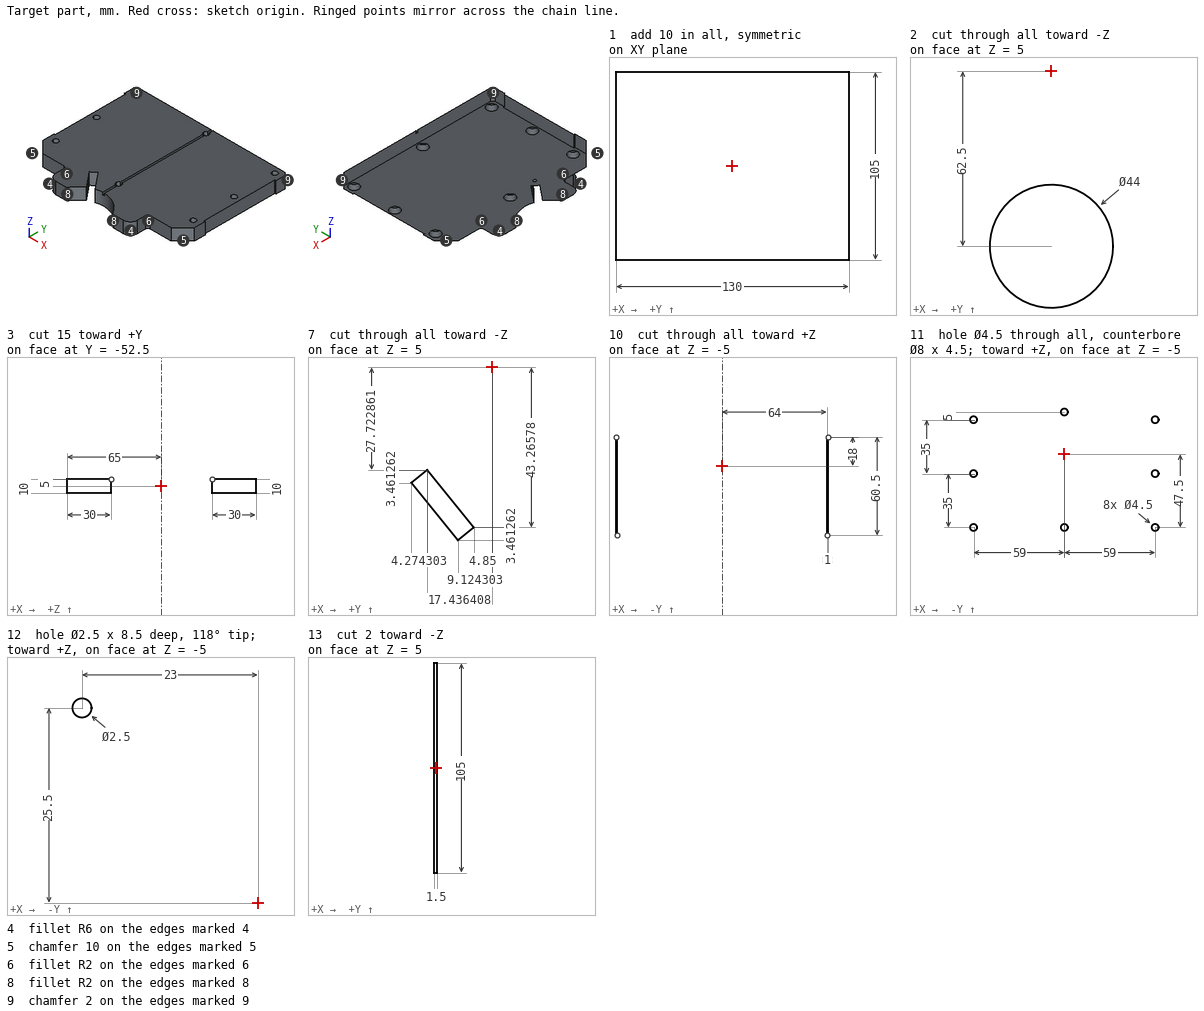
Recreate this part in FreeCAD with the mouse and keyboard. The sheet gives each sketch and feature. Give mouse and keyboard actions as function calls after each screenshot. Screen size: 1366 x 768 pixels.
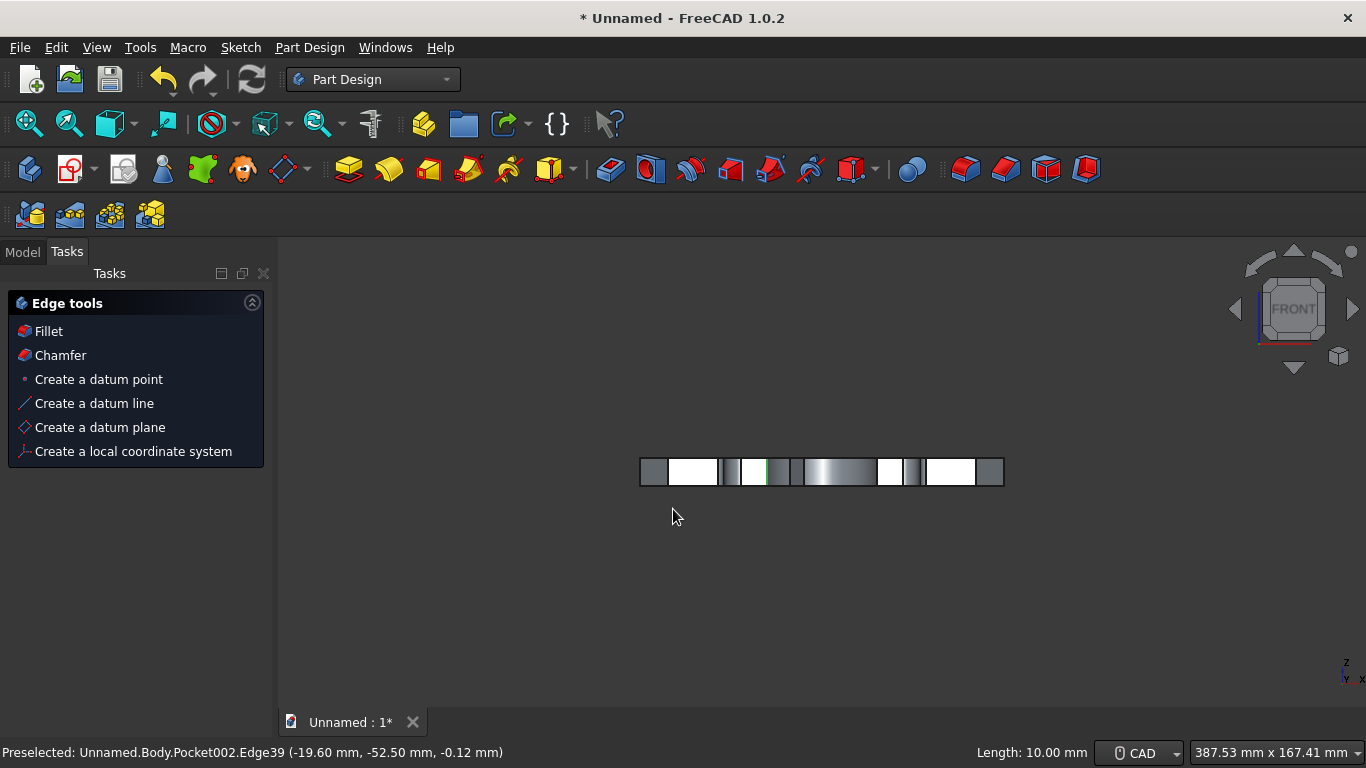
click(30, 124)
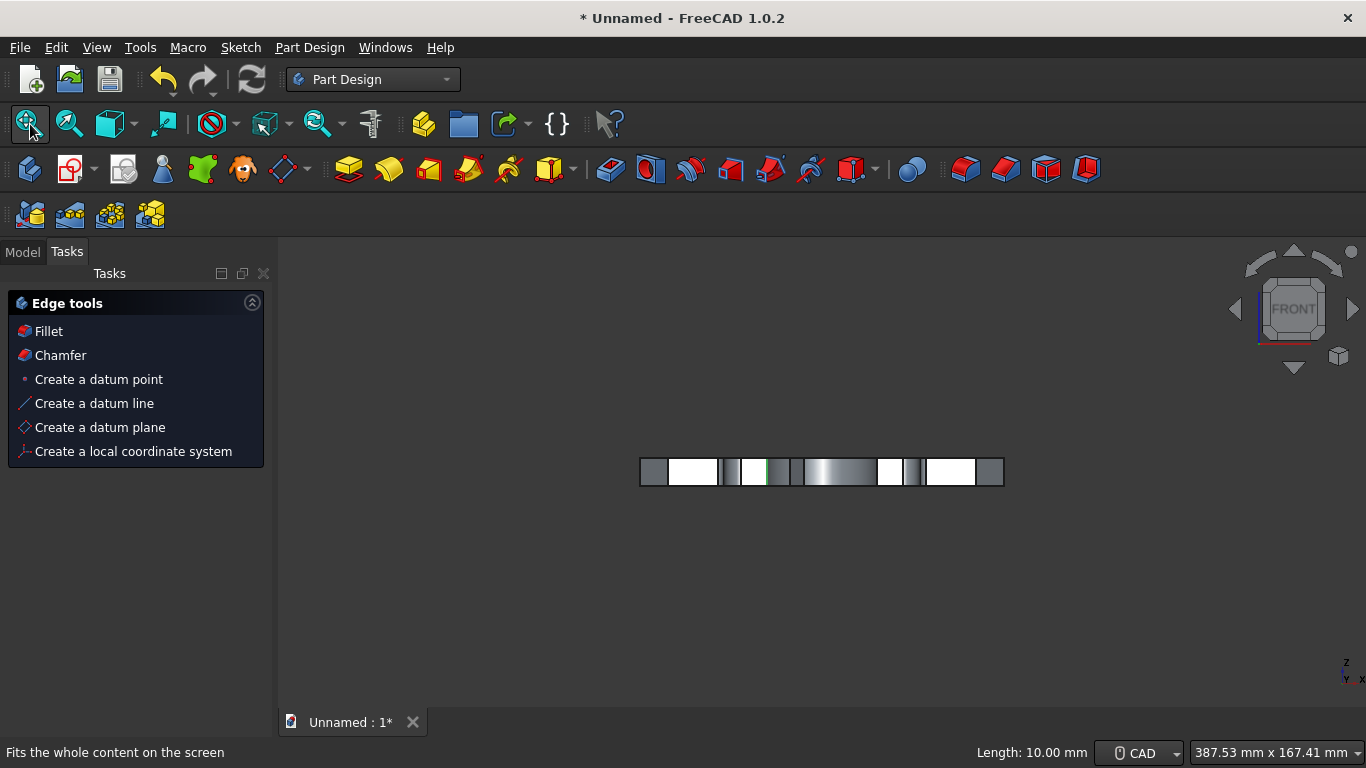
click(877, 471, ctrl)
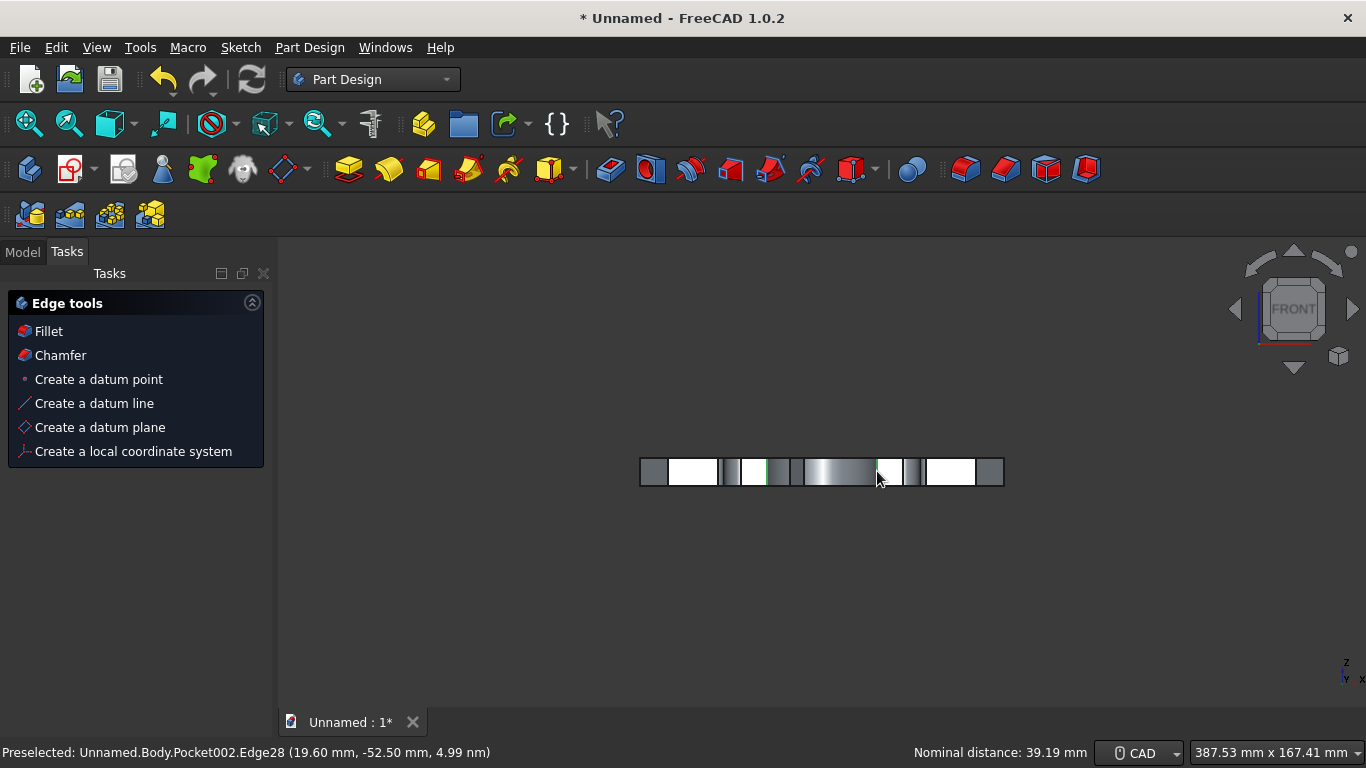
click(966, 170)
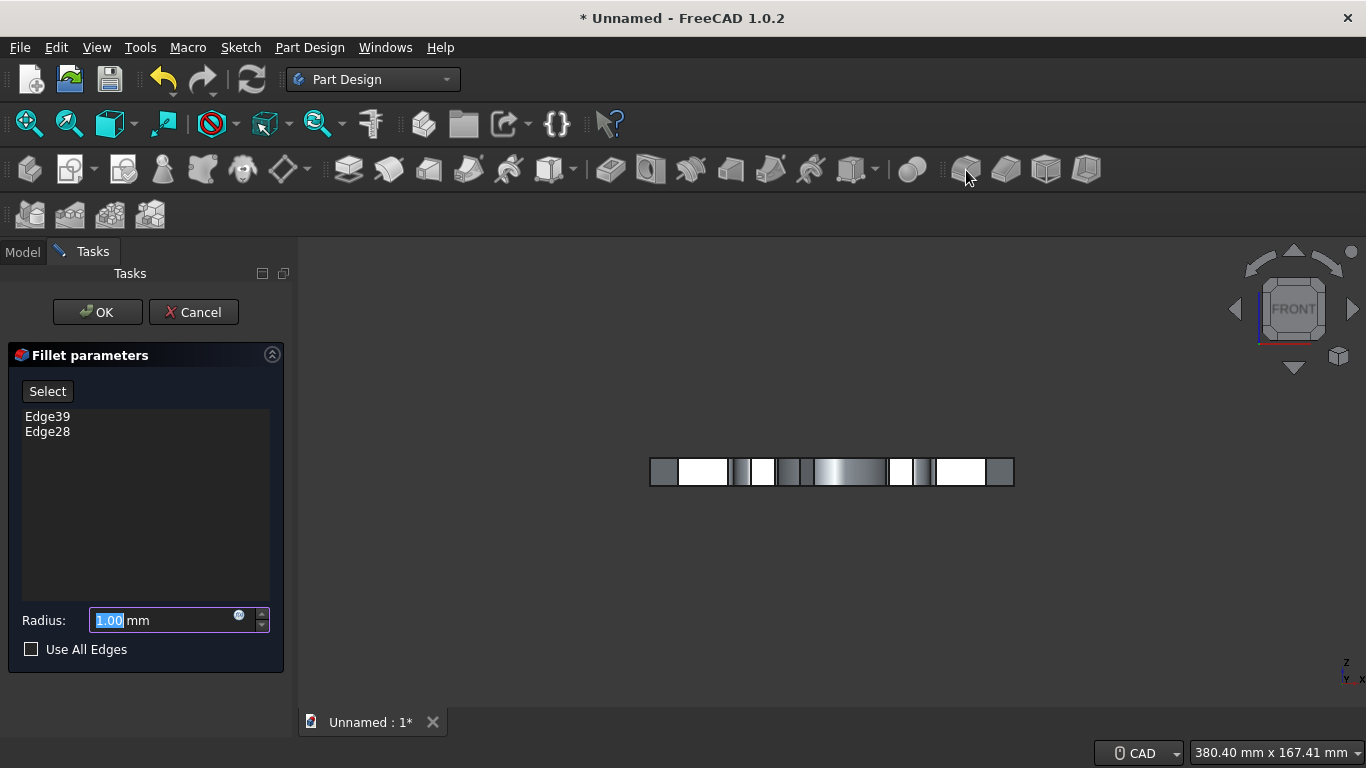
text(2)
key(Tab)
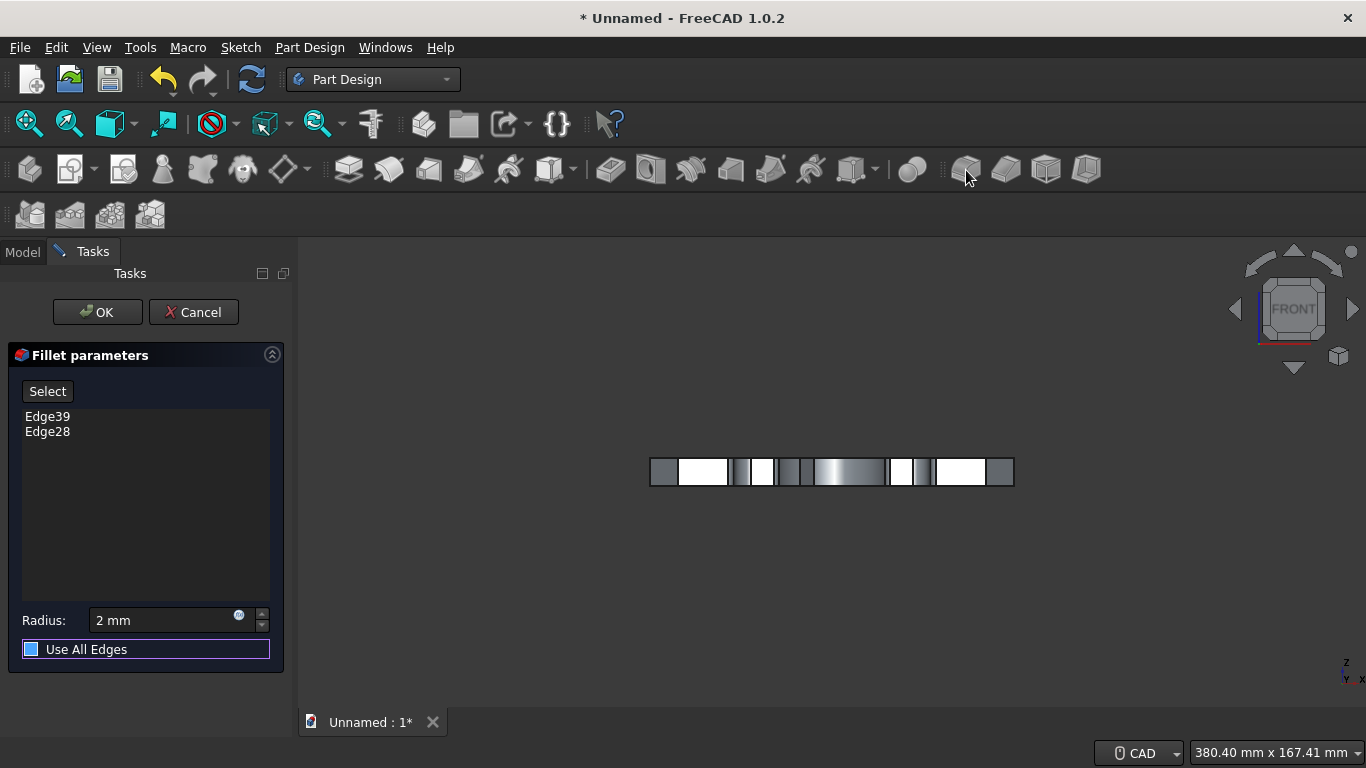
click(98, 312)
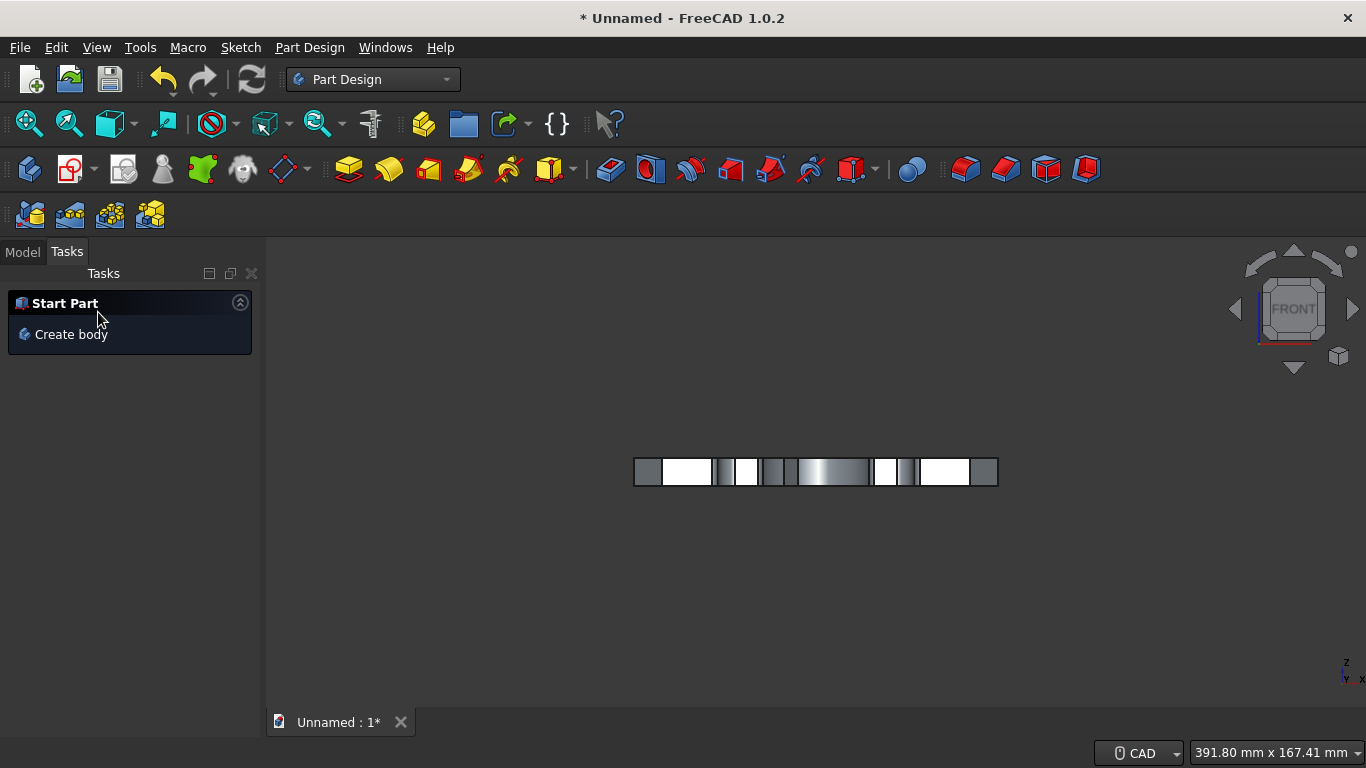
click(30, 124)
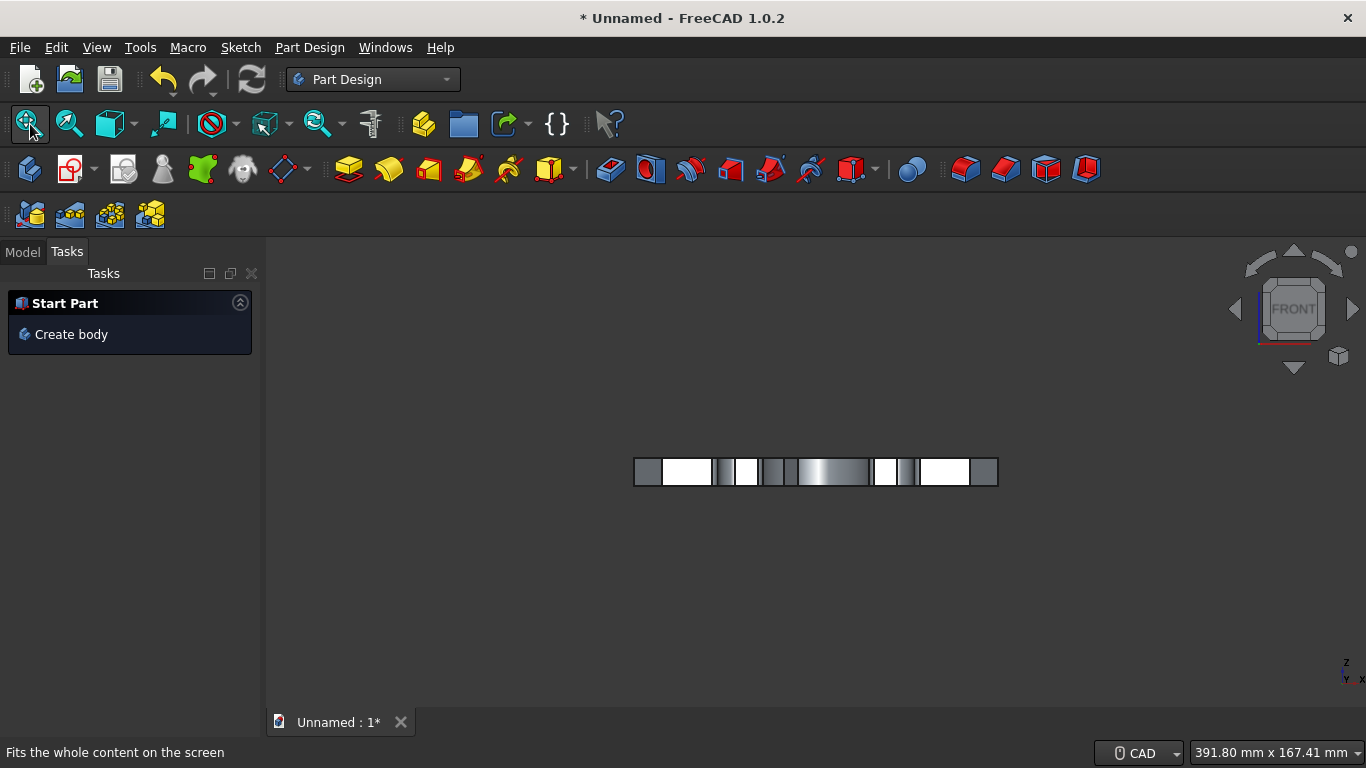
key(0)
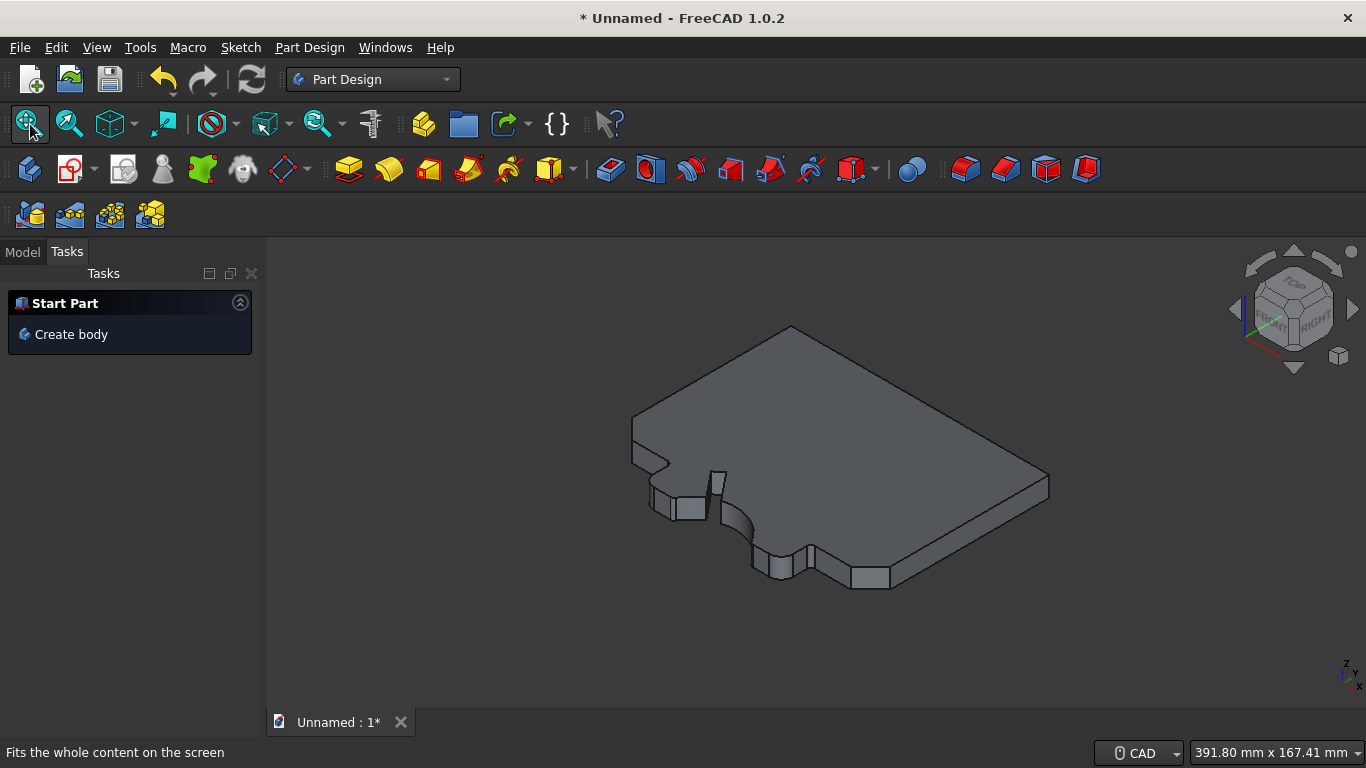
key(2)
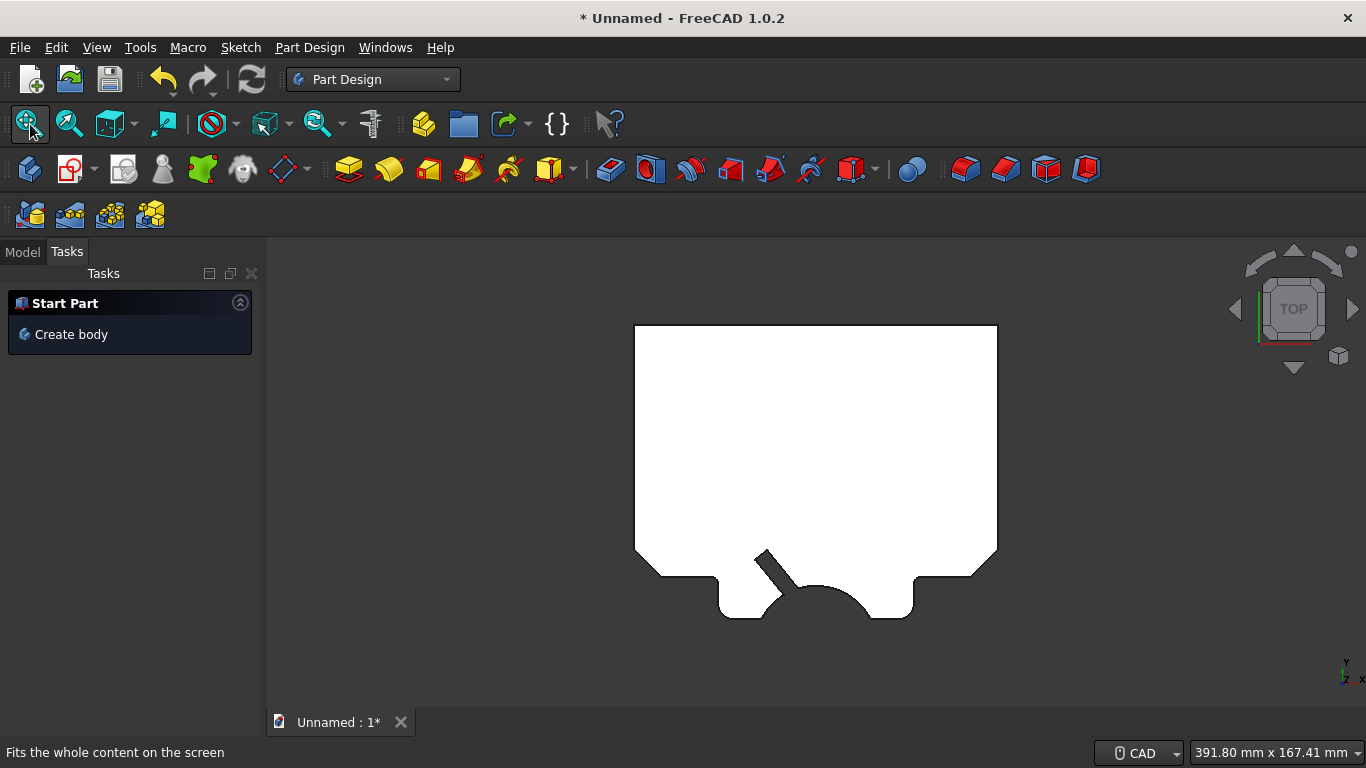
key(1)